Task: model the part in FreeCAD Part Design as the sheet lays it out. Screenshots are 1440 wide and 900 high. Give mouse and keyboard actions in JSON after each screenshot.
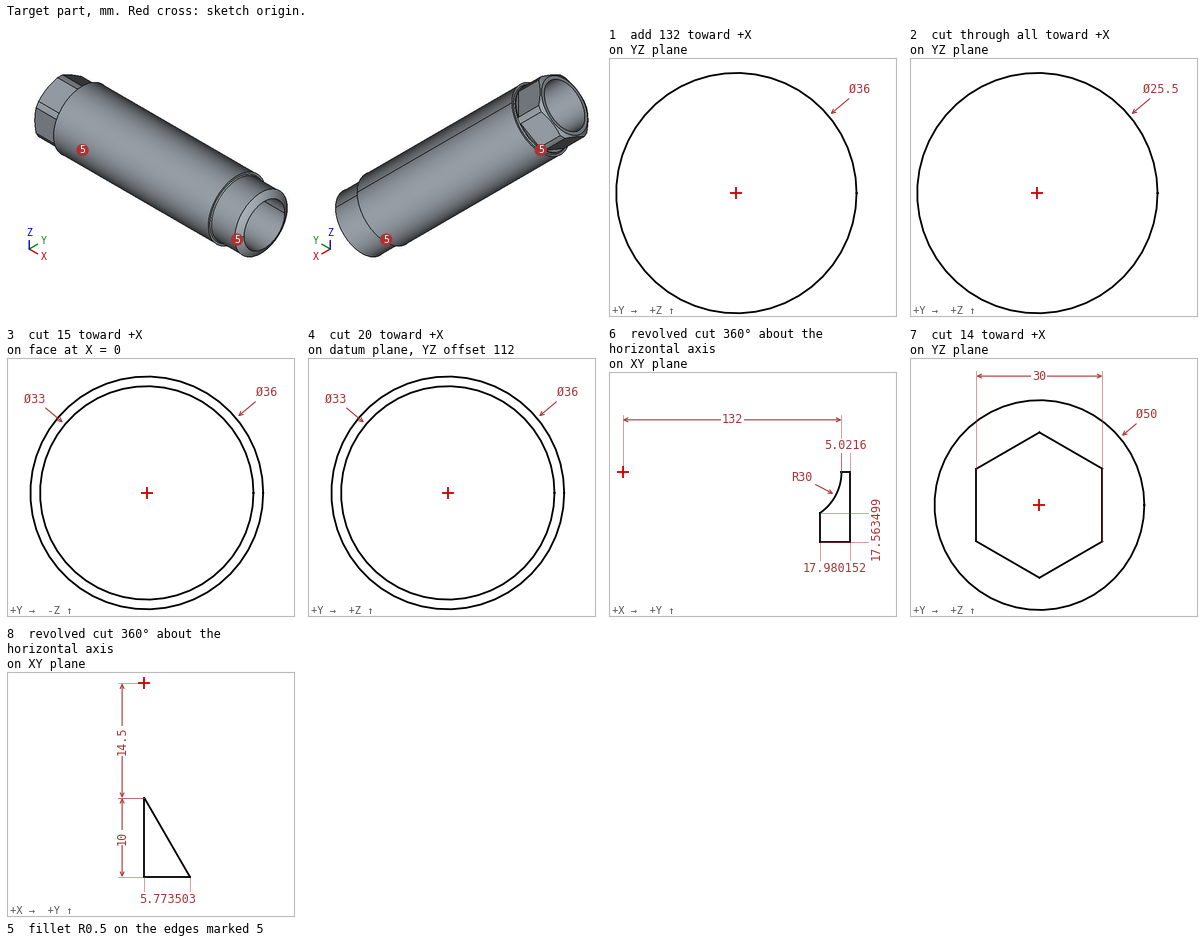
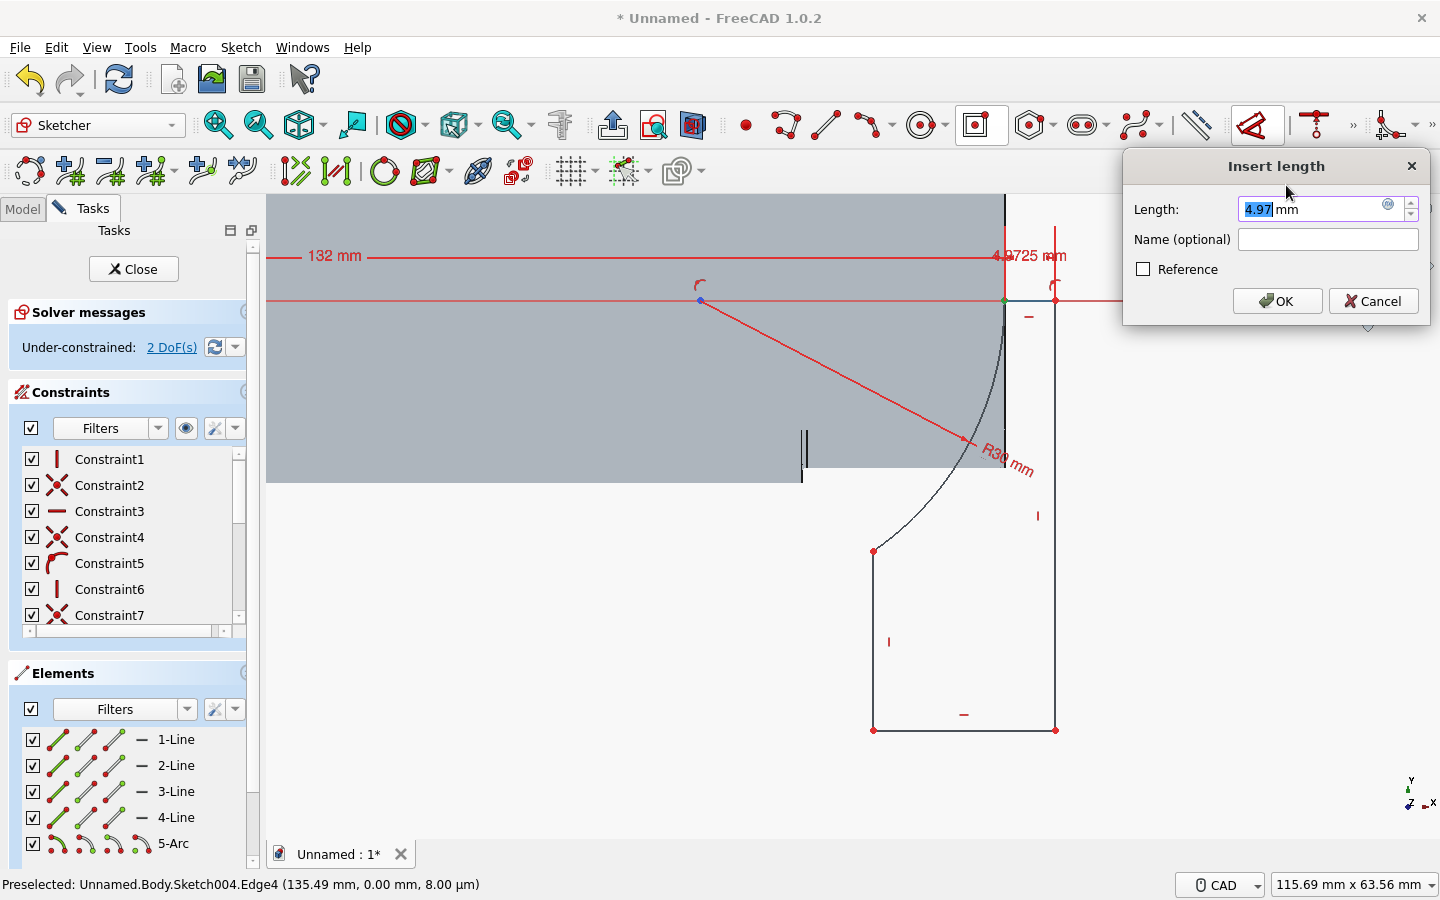
{"action": "type", "text": "5.0216"}
{"action": "key", "text": "Return"}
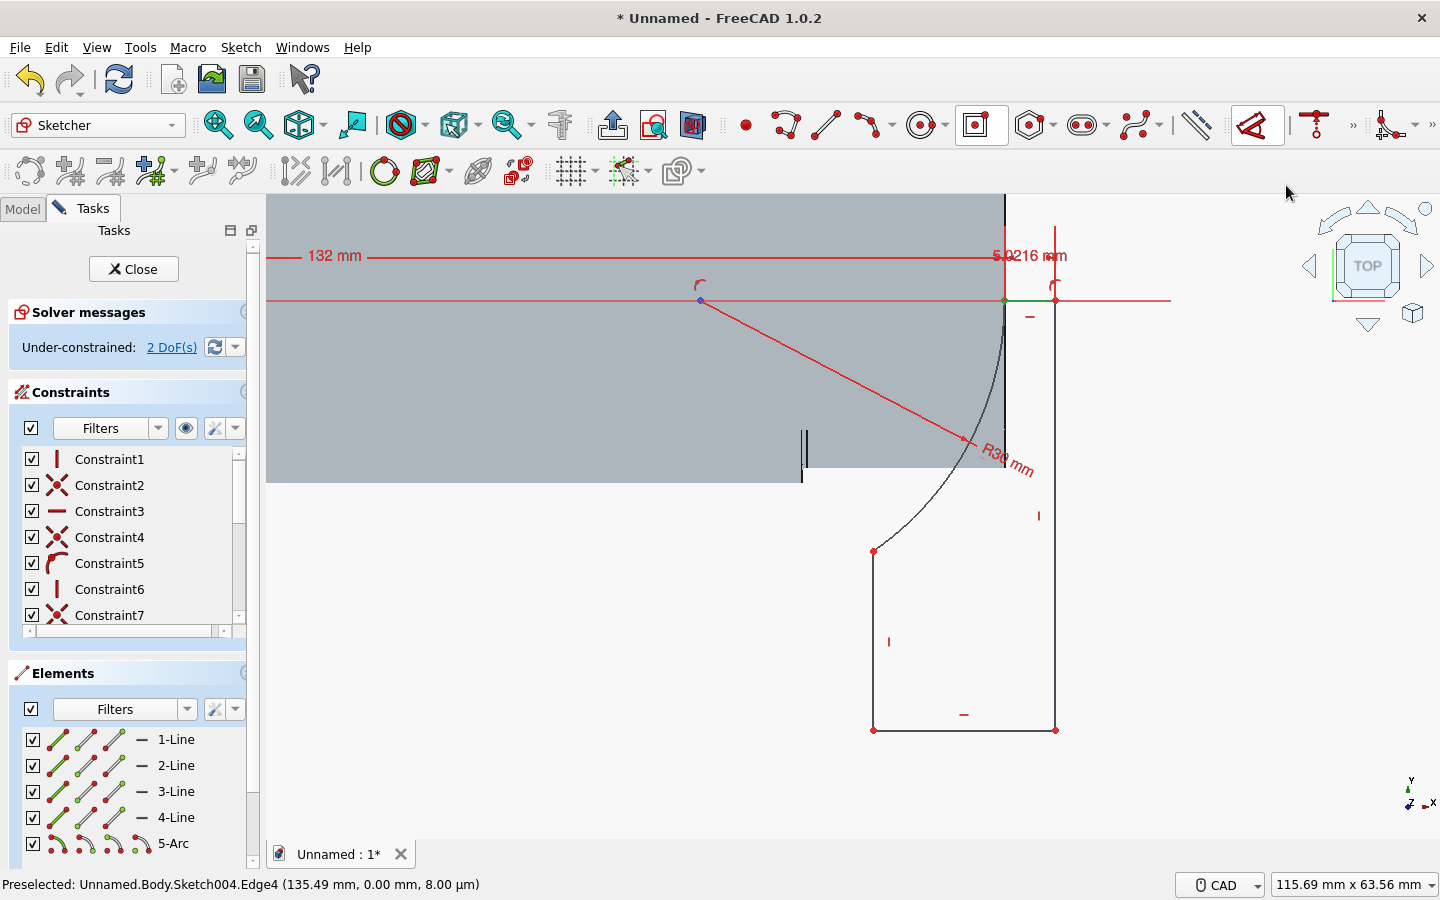
{"action": "left_click", "coordinate": [873, 605]}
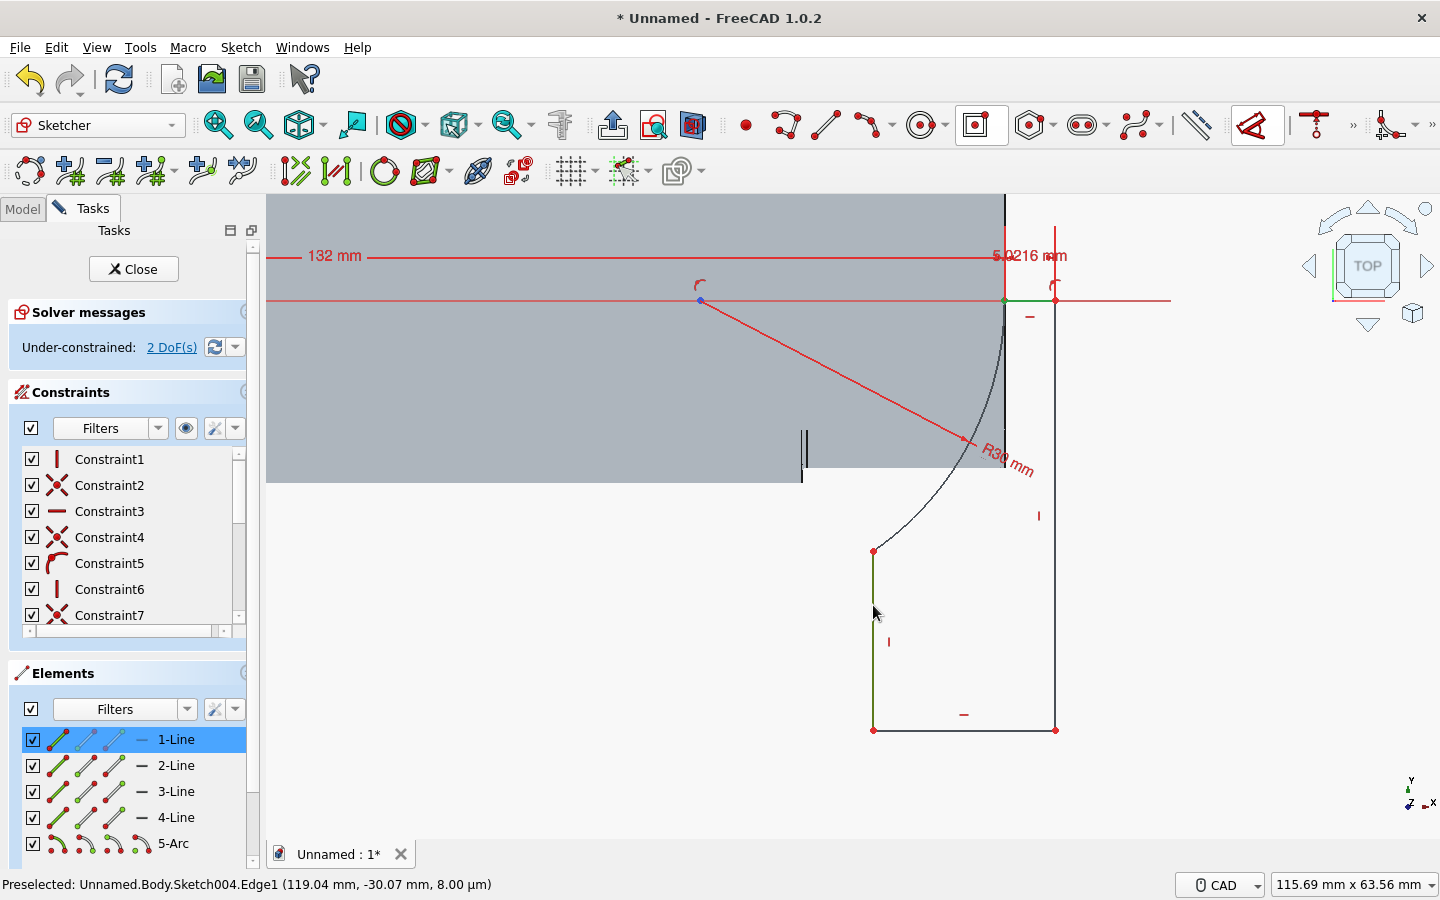
{"action": "key", "text": "i"}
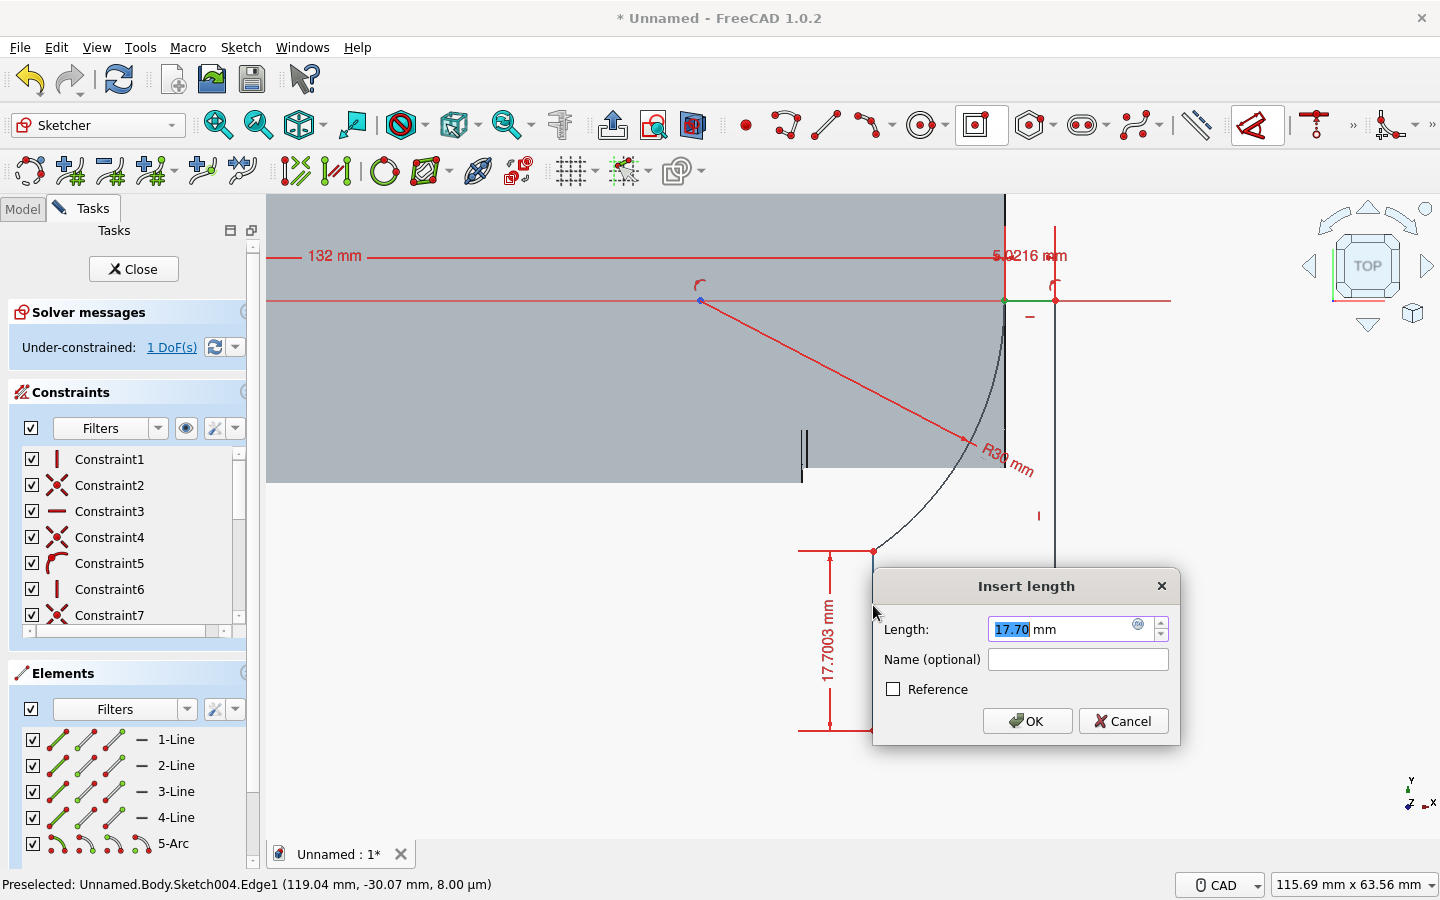
{"action": "type", "text": "17.563499"}
{"action": "key", "text": "Return"}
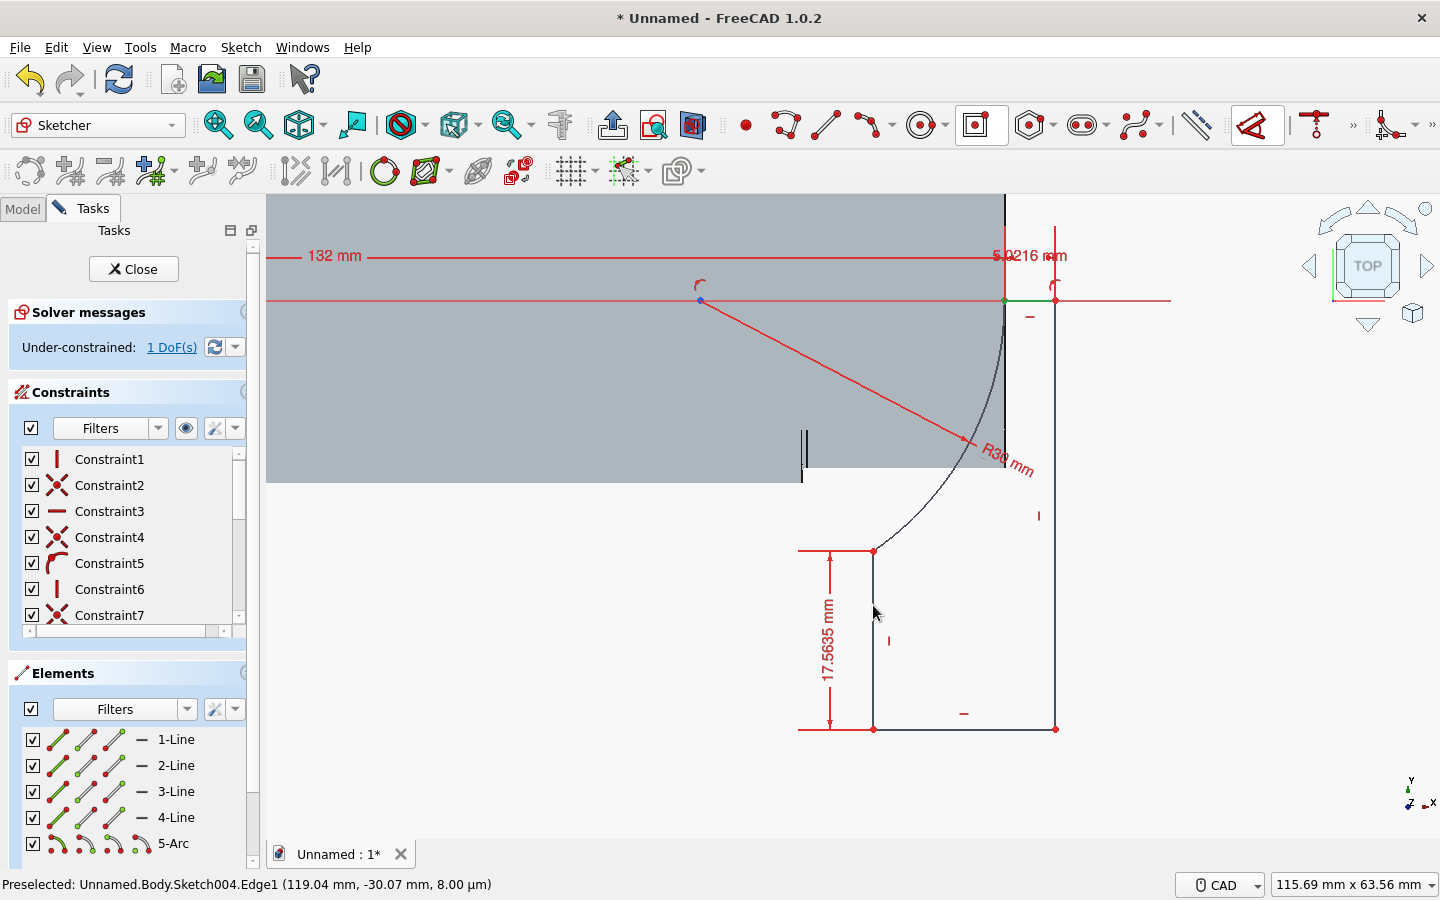
{"action": "left_click", "coordinate": [928, 730]}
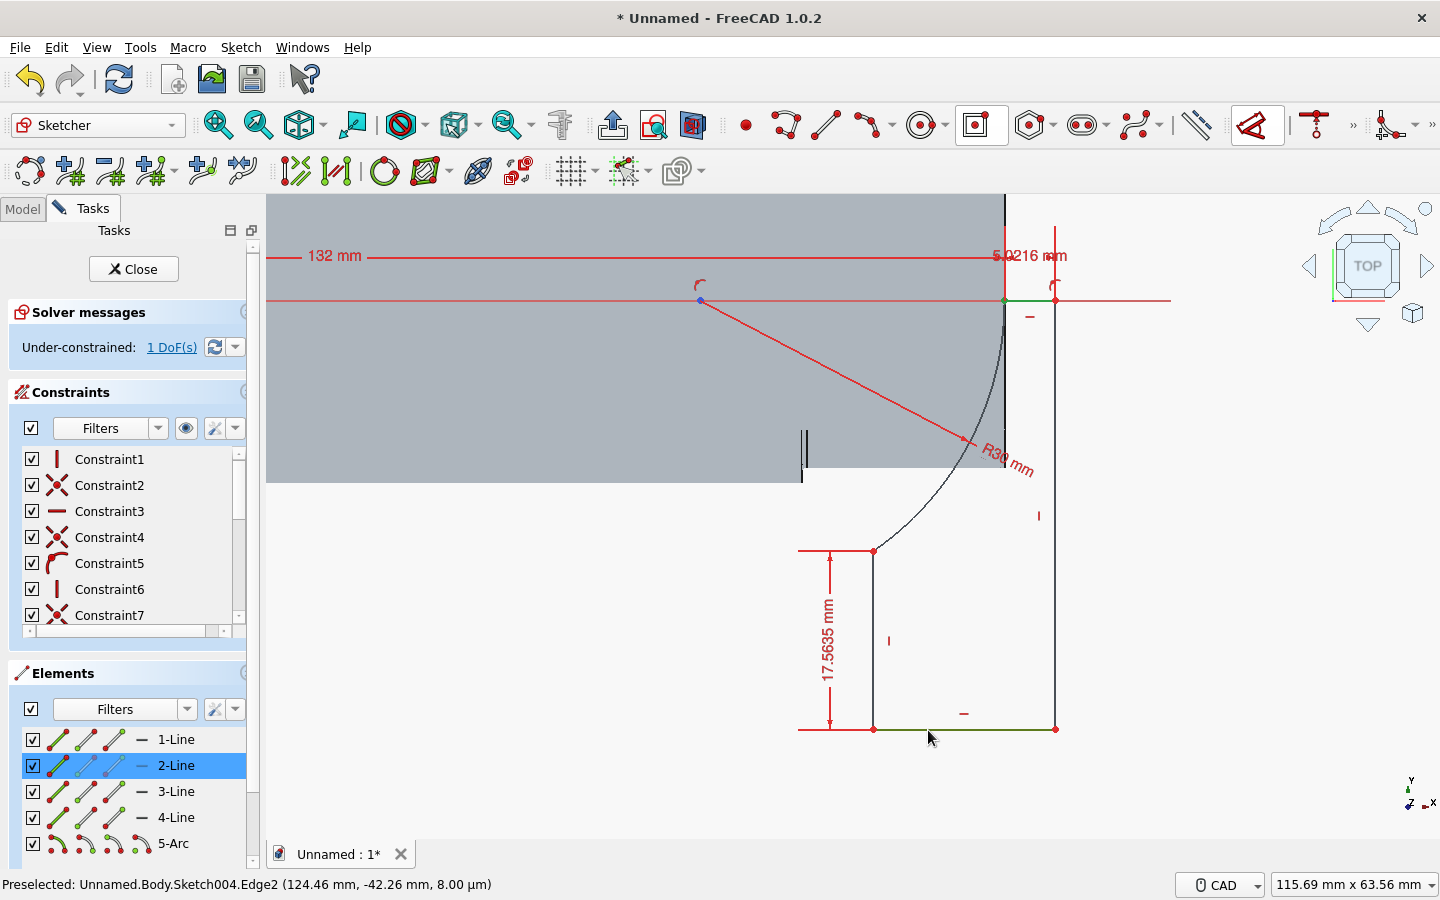
{"action": "left_click", "coordinate": [1278, 126]}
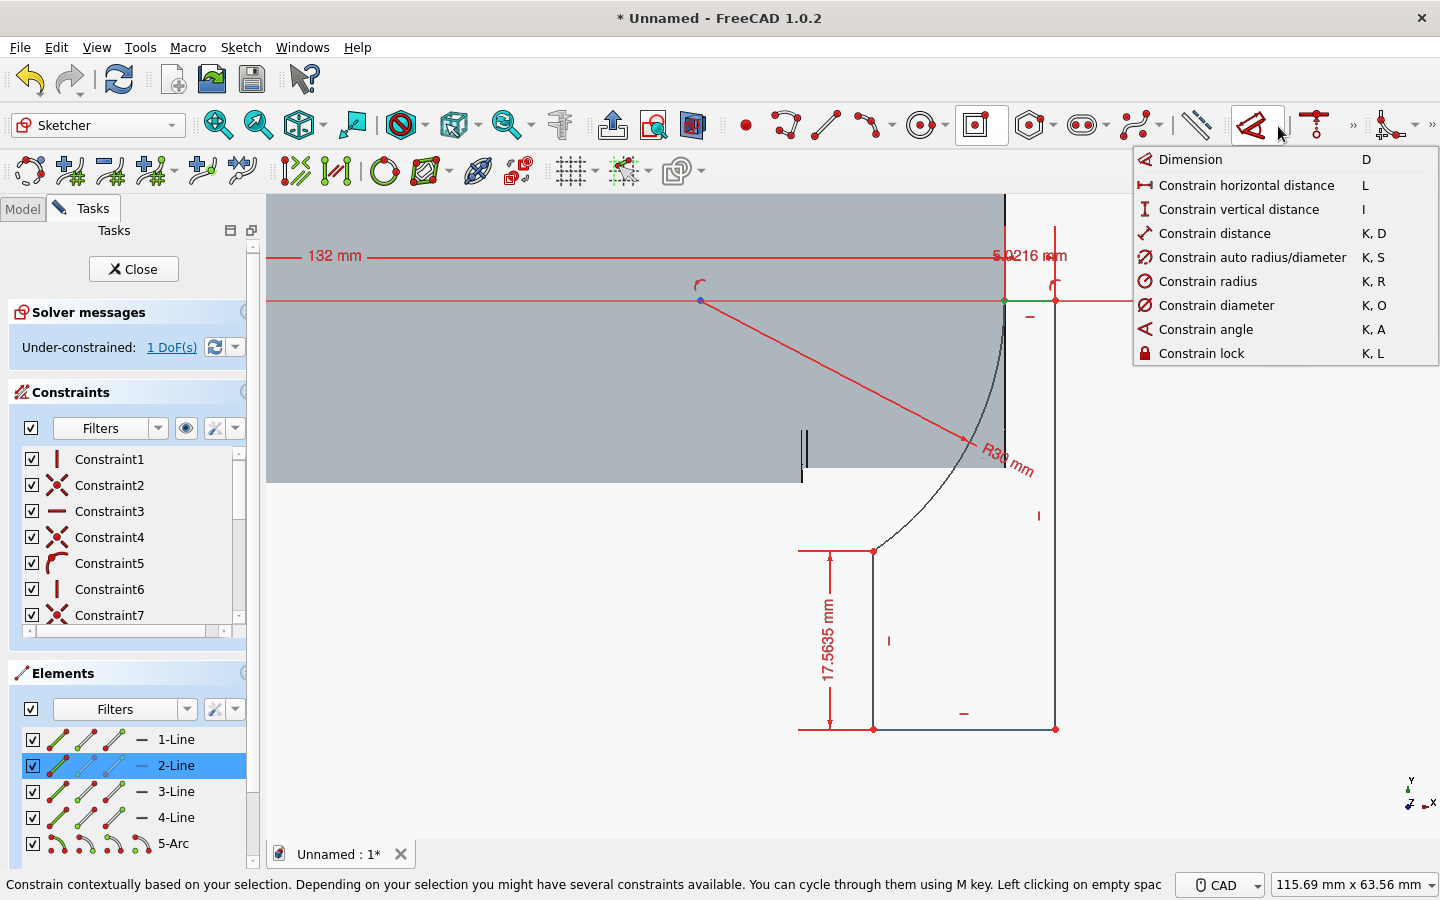
{"action": "left_click", "coordinate": [1286, 185]}